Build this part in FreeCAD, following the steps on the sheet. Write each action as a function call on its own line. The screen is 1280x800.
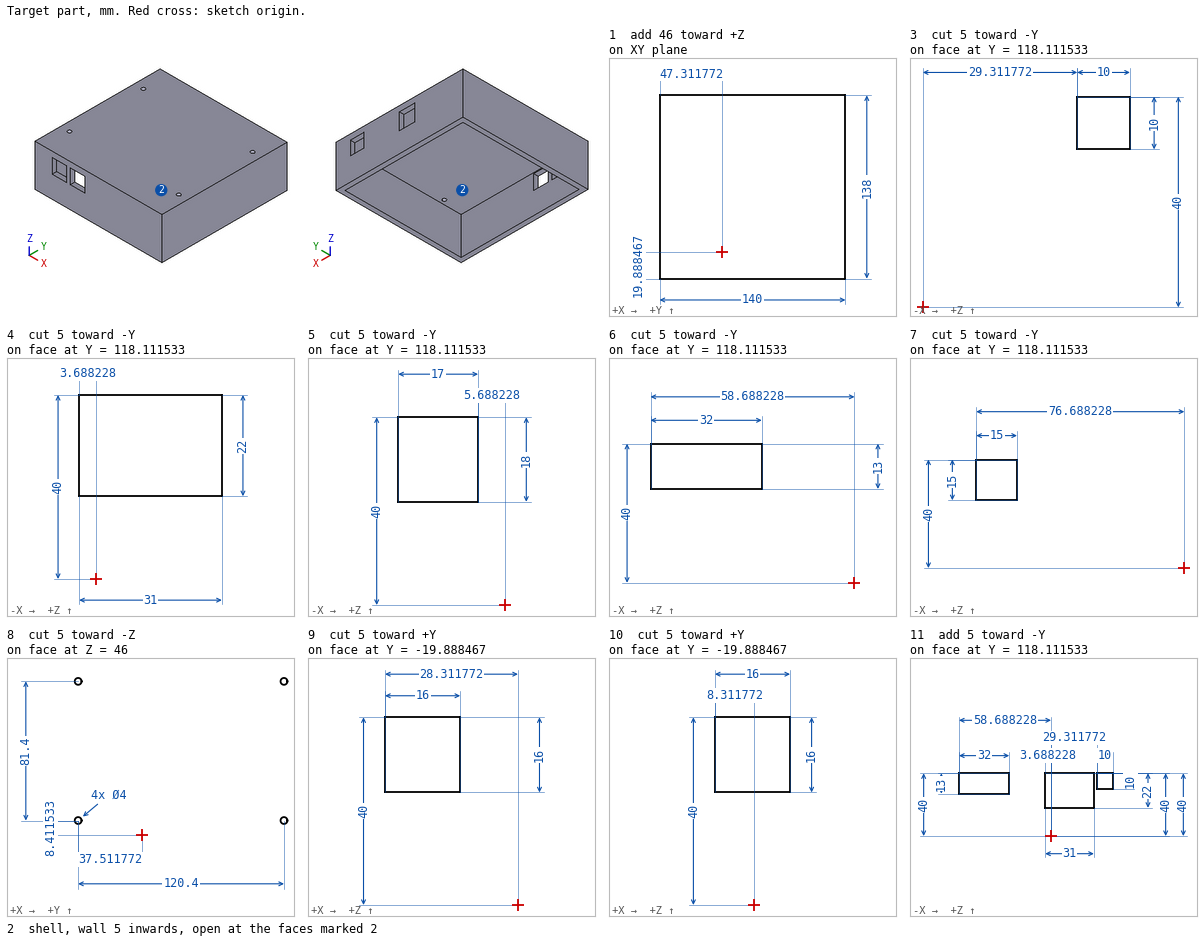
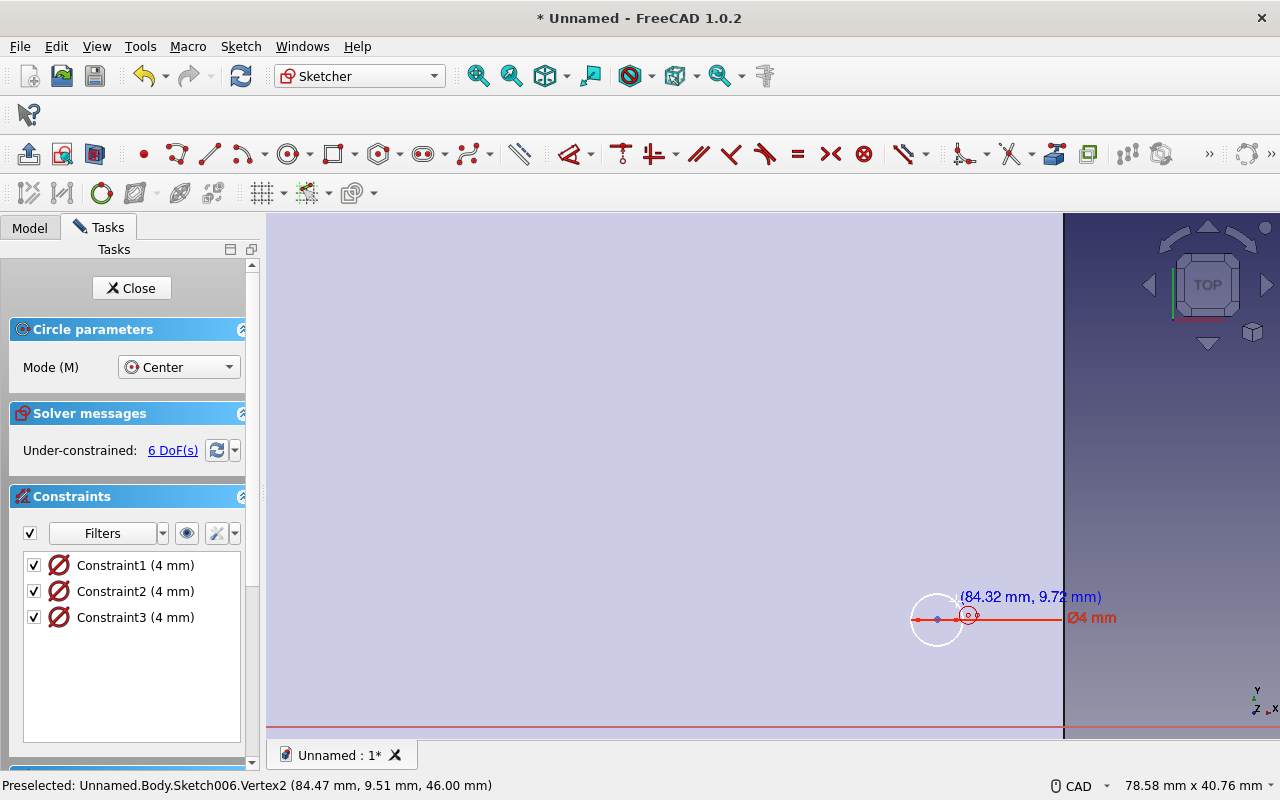
scroll(939, 623, down, 6)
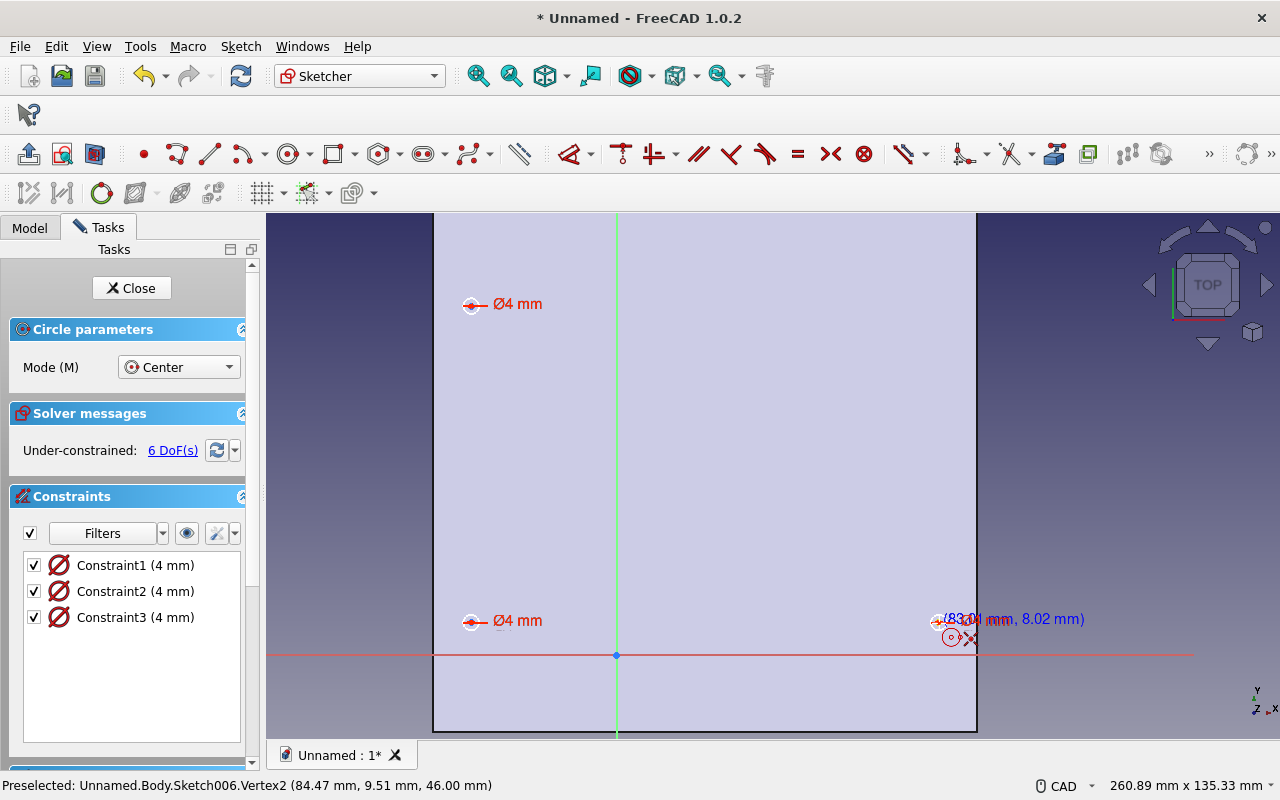
scroll(939, 306, up, 6)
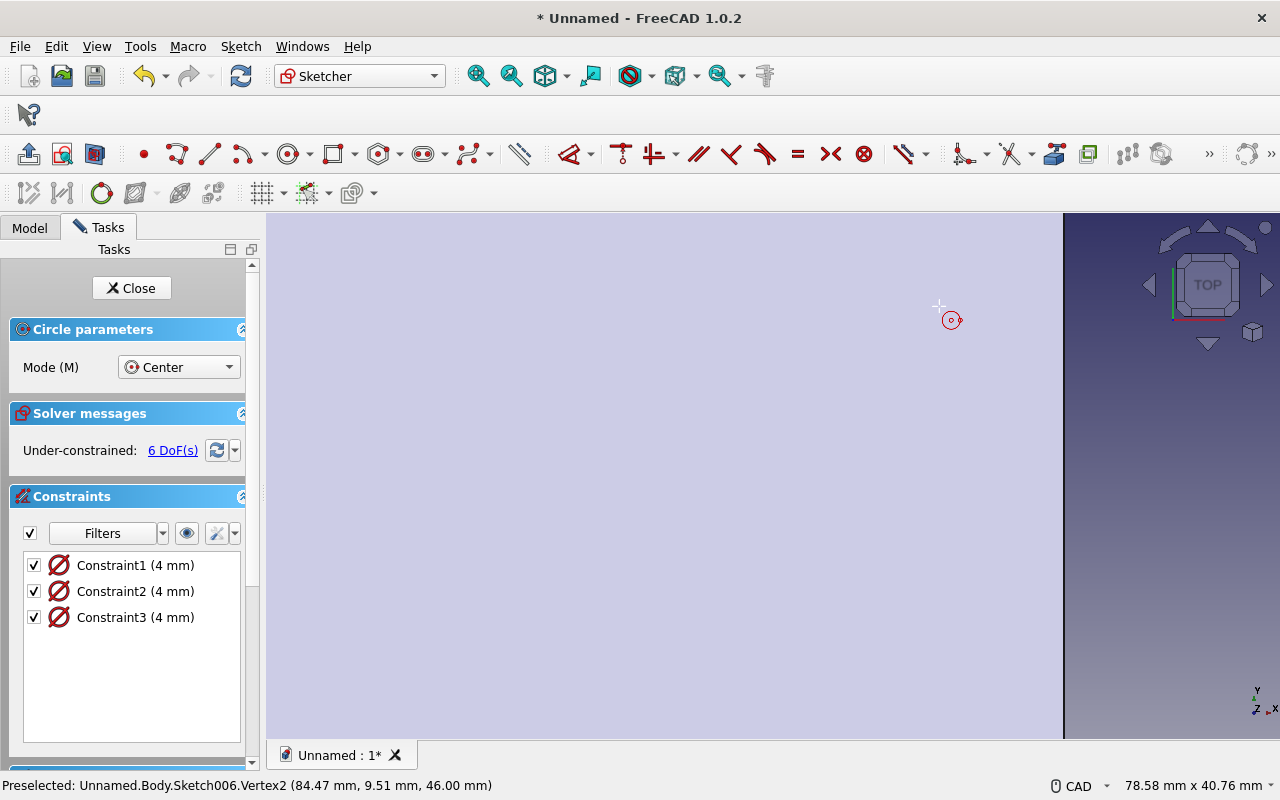
click(937, 305)
move(956, 287)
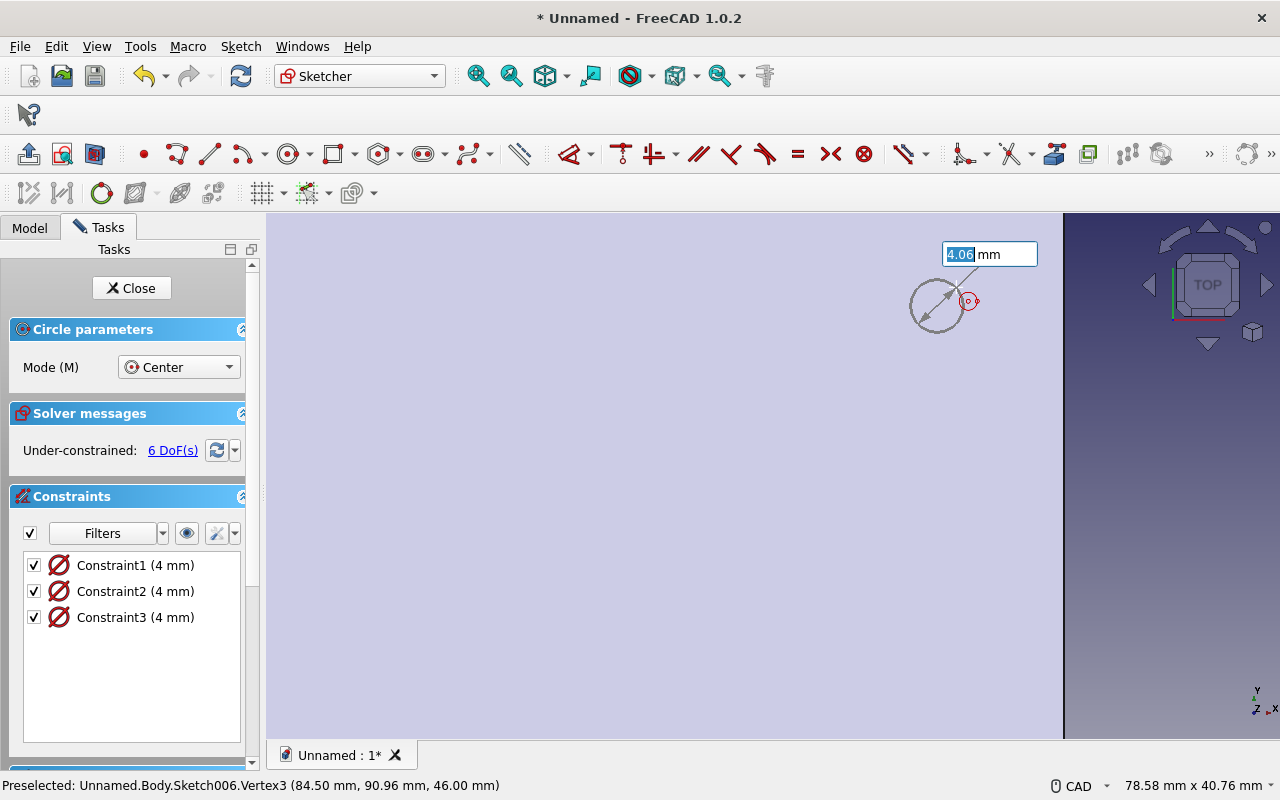
text(4)
key(Return)
key(Escape)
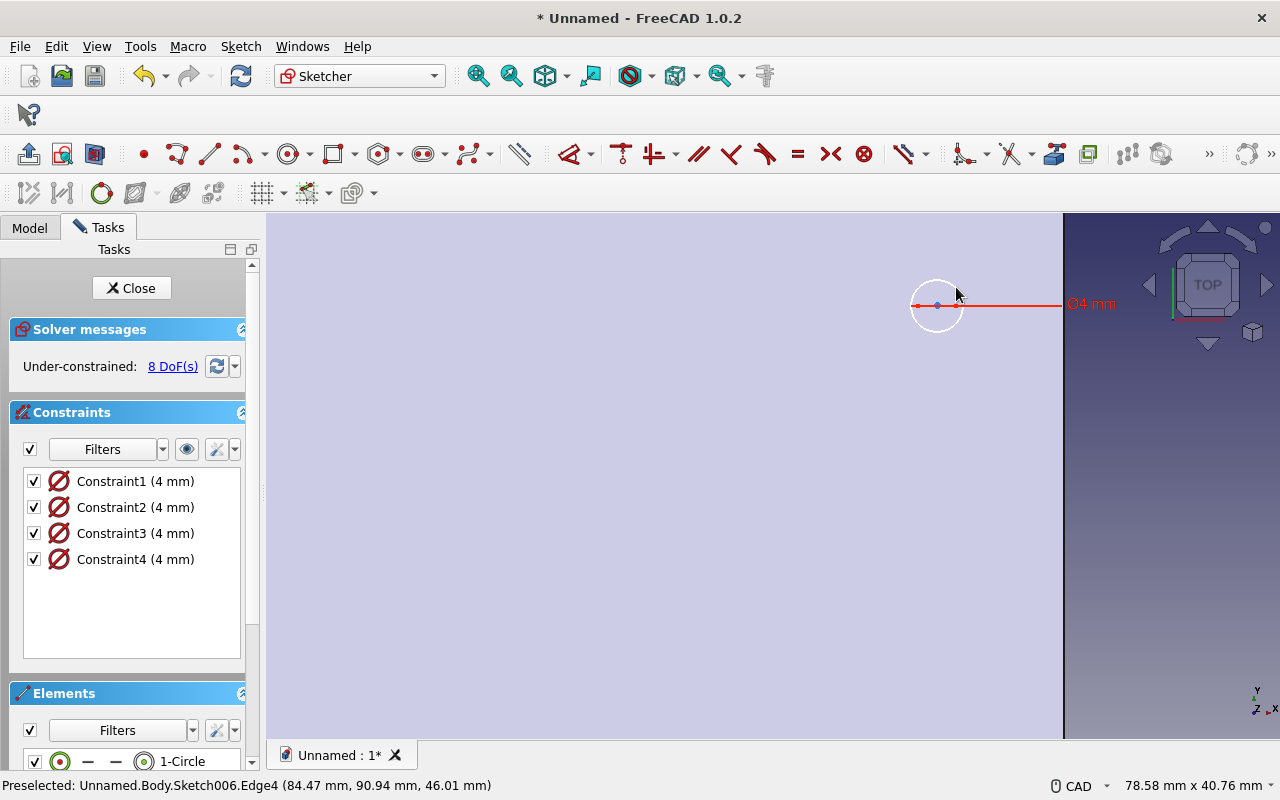
scroll(939, 305, down, 6)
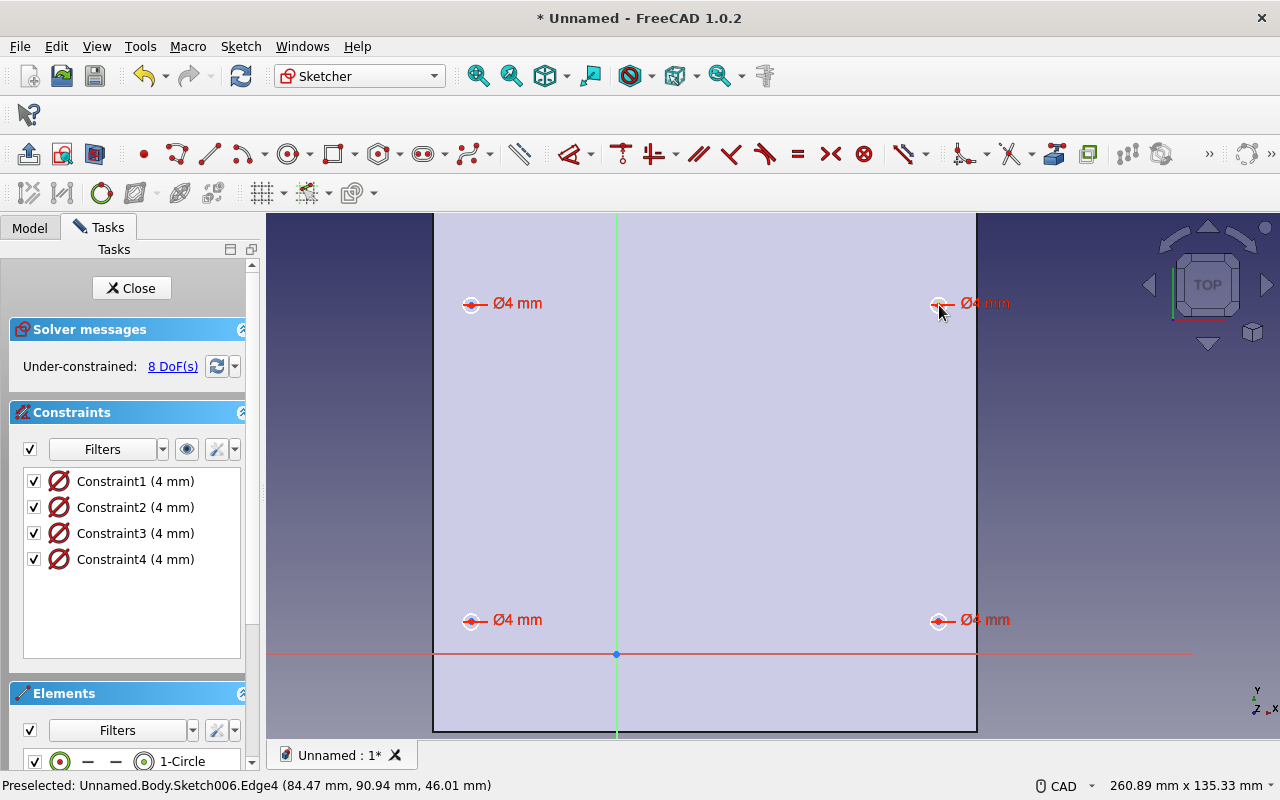
click(471, 622)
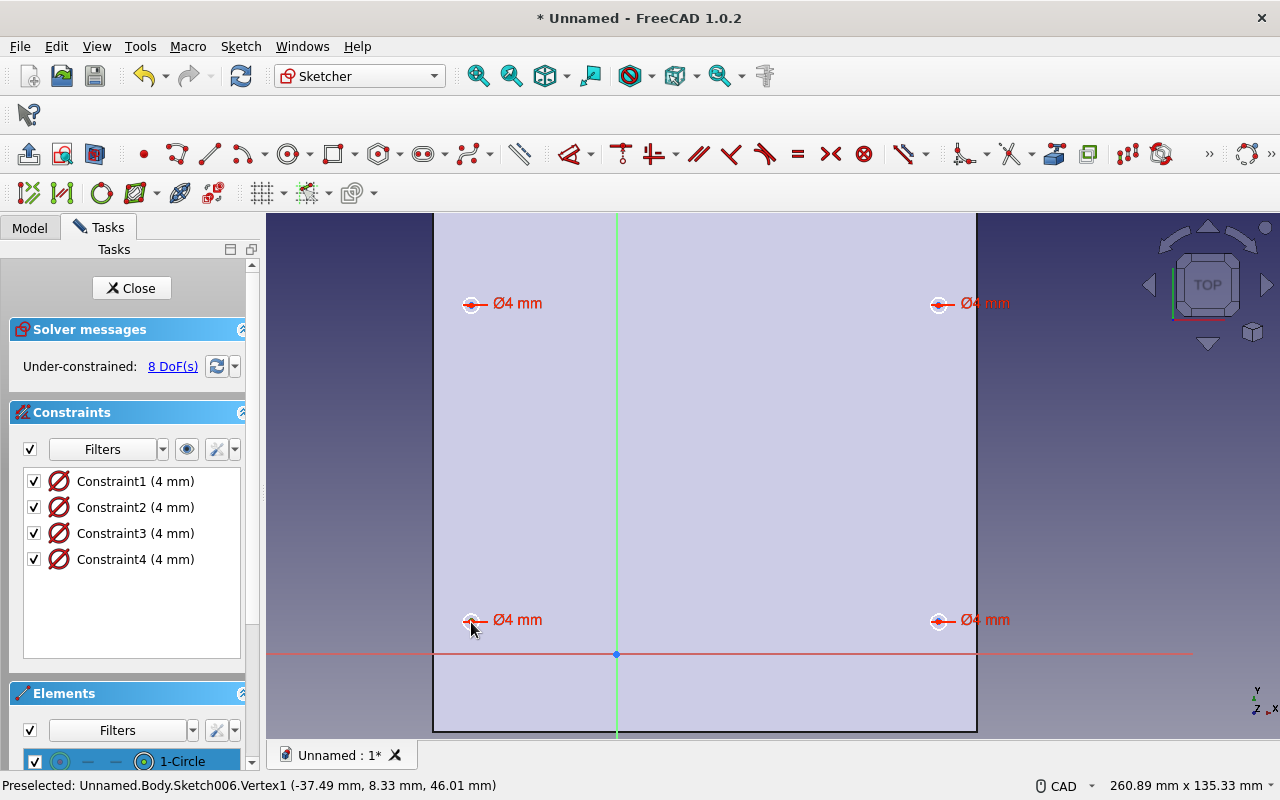
click(471, 305)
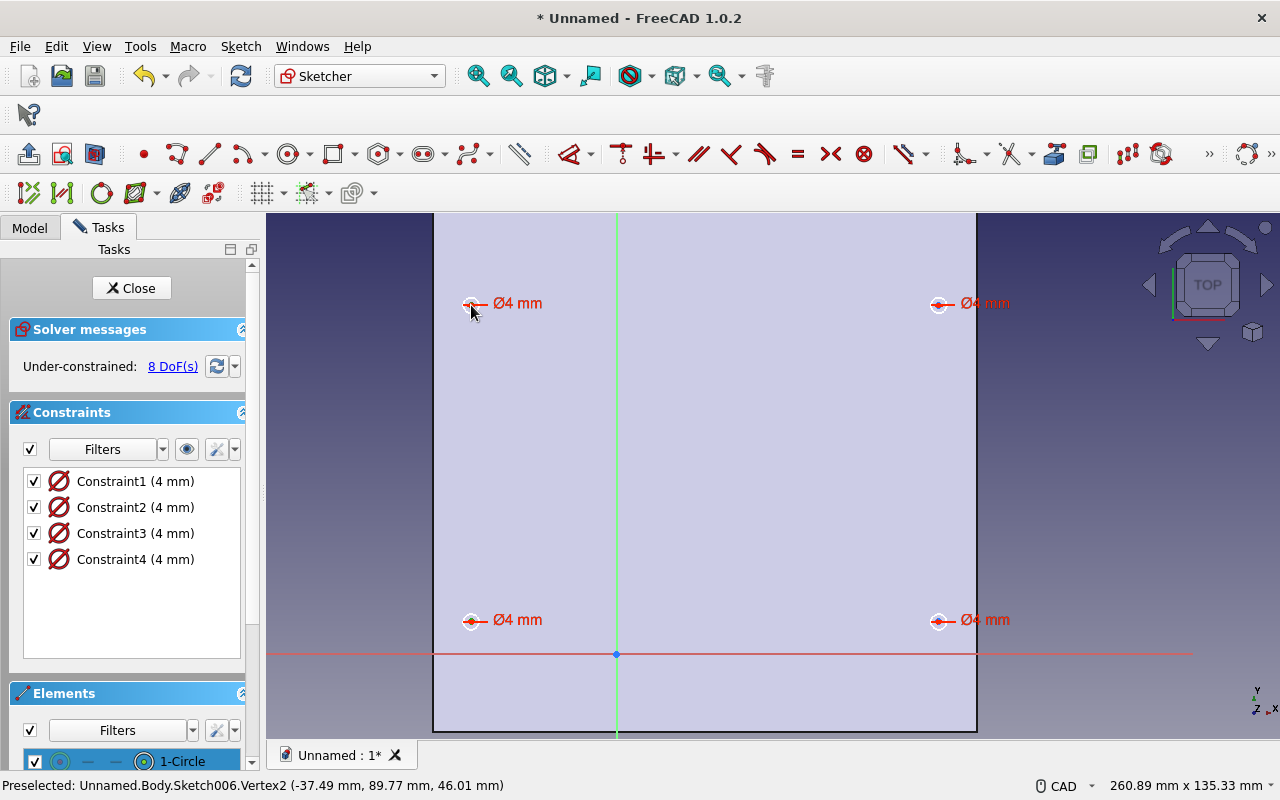
key(v)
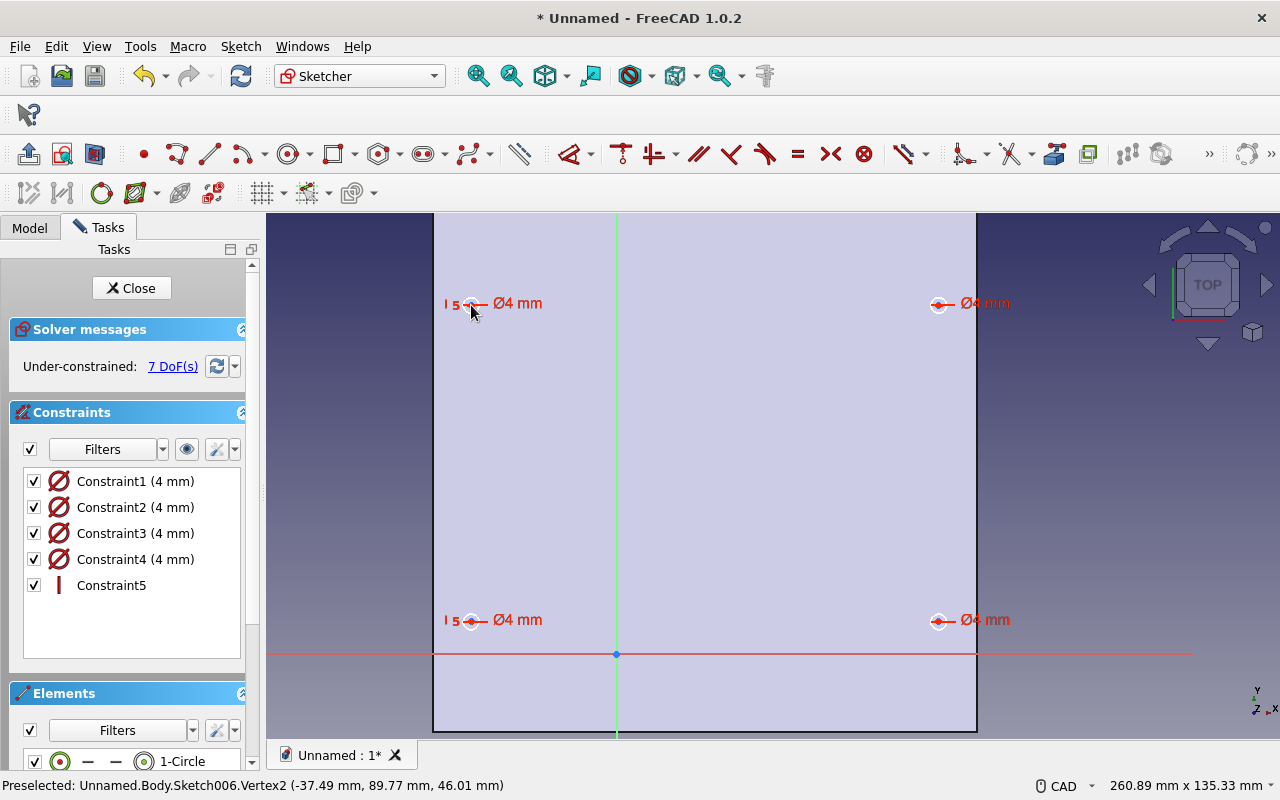
click(471, 622)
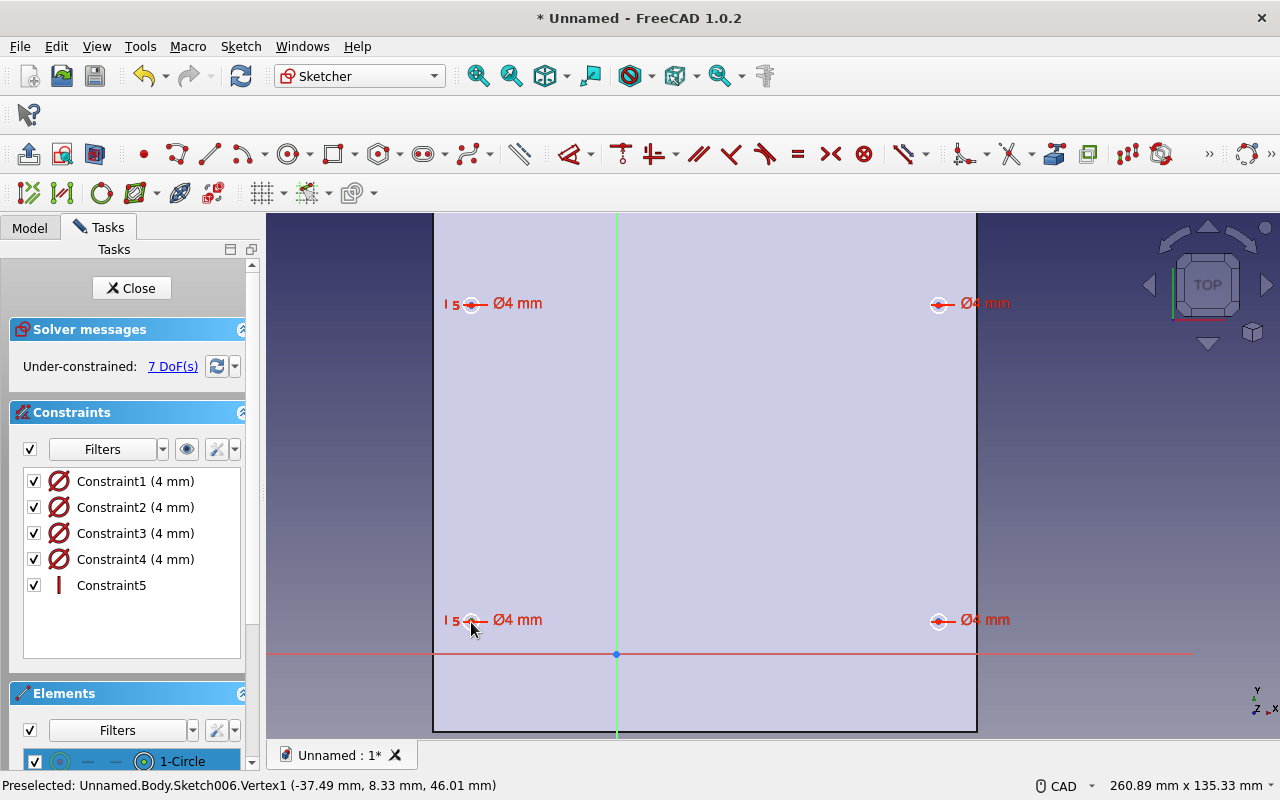
click(939, 622)